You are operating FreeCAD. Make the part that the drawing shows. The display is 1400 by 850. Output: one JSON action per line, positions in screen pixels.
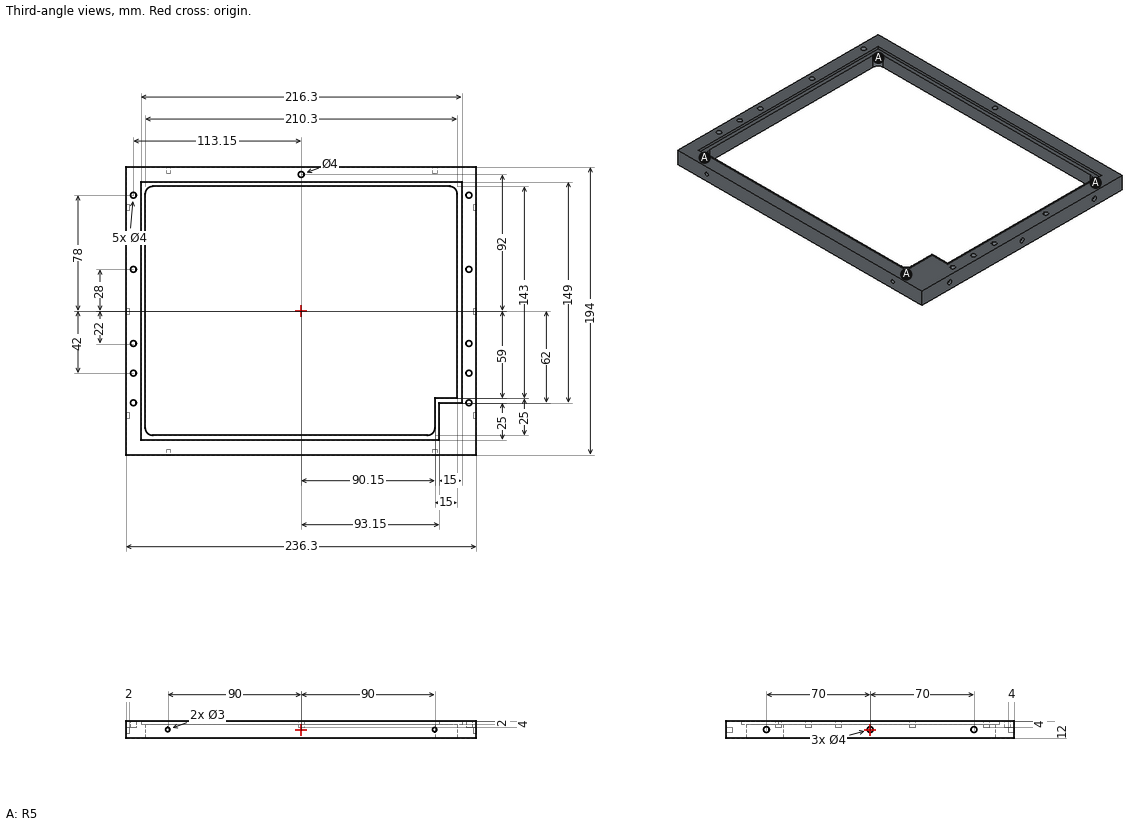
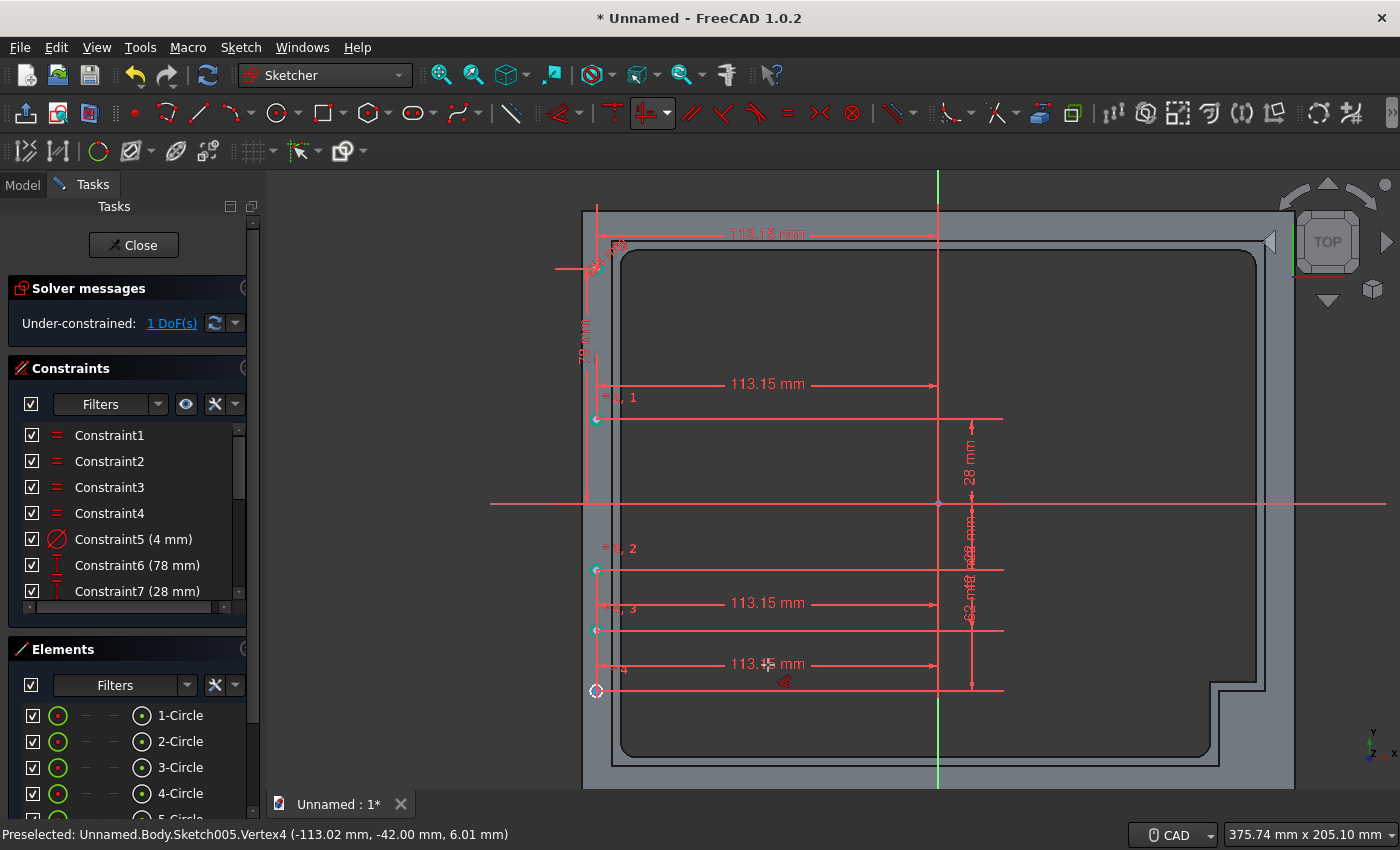
{"action": "left_click", "coordinate": [596, 691]}
{"action": "left_click", "coordinate": [767, 725]}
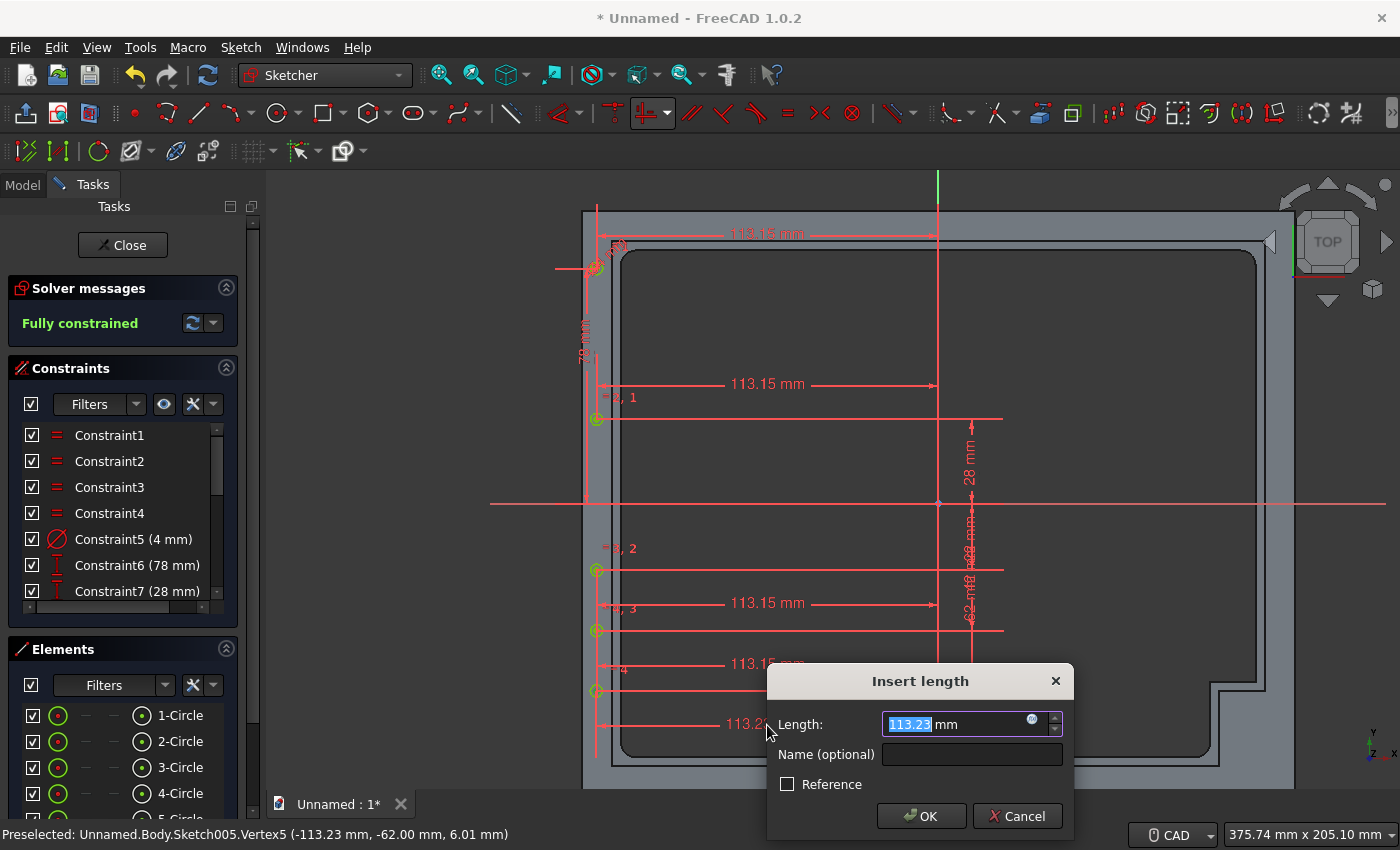
{"action": "type", "text": "113.15"}
{"action": "key", "text": "Return"}
{"action": "key", "text": "Escape"}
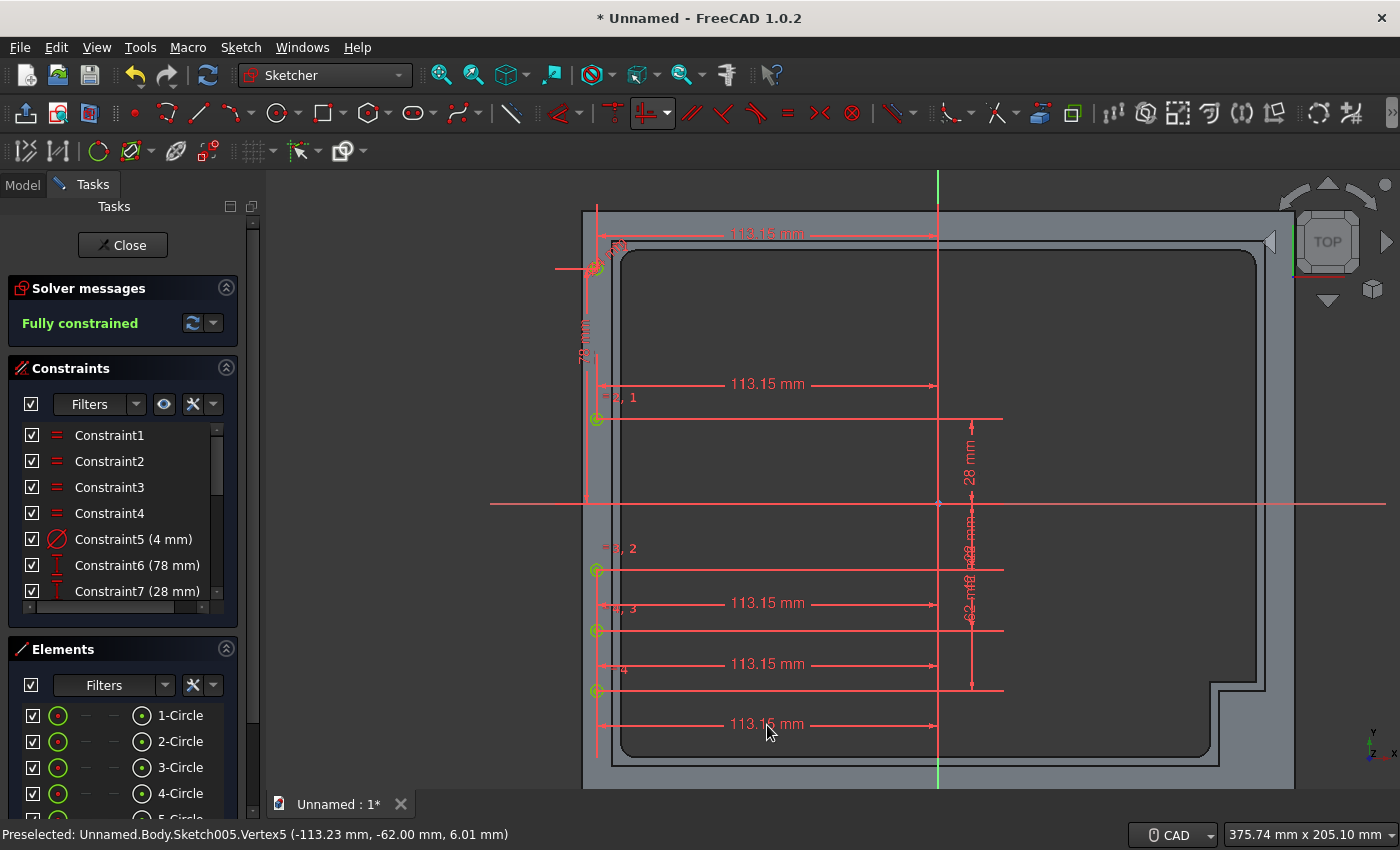
{"action": "left_click", "coordinate": [123, 245]}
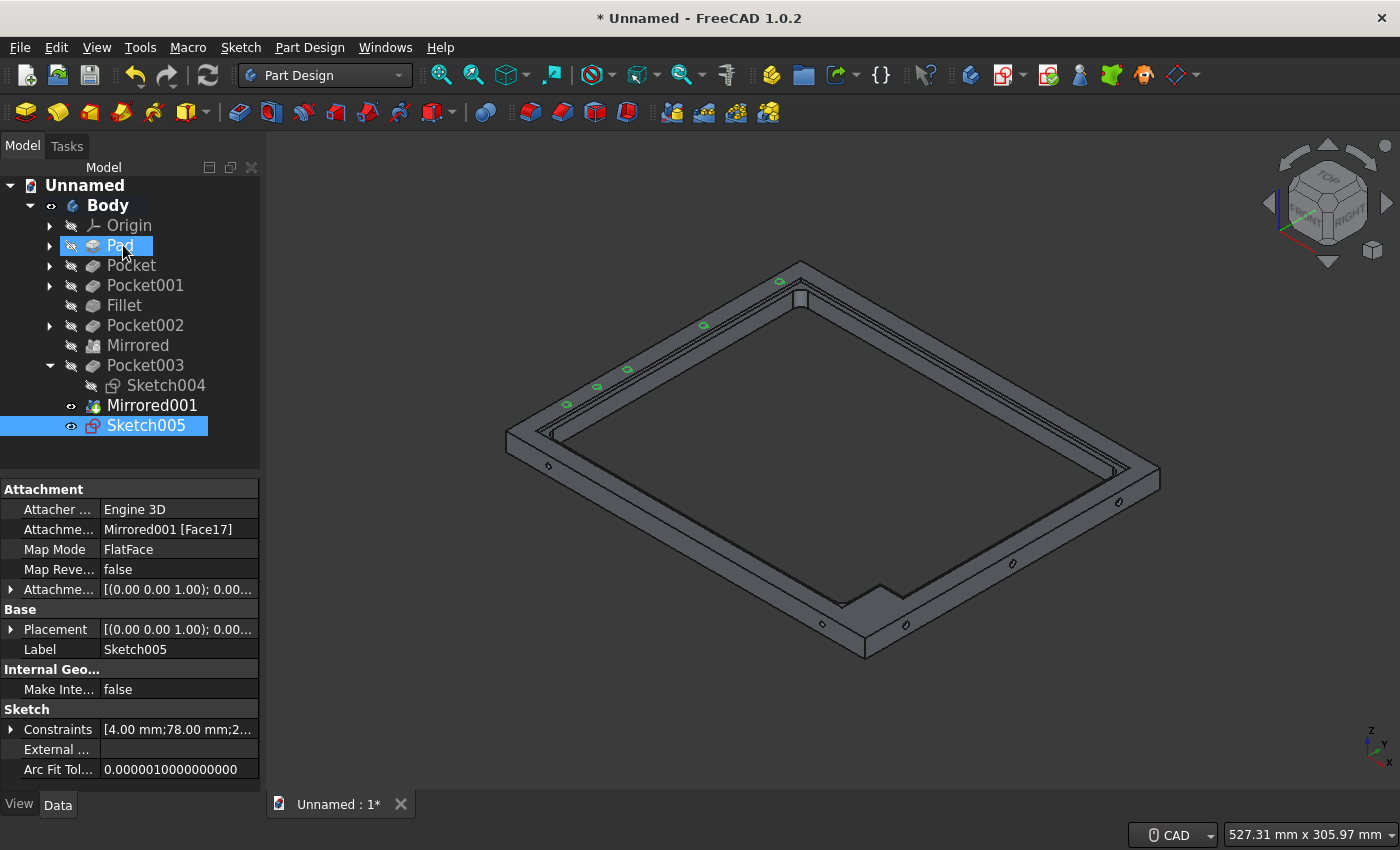
{"action": "left_click", "coordinate": [240, 112]}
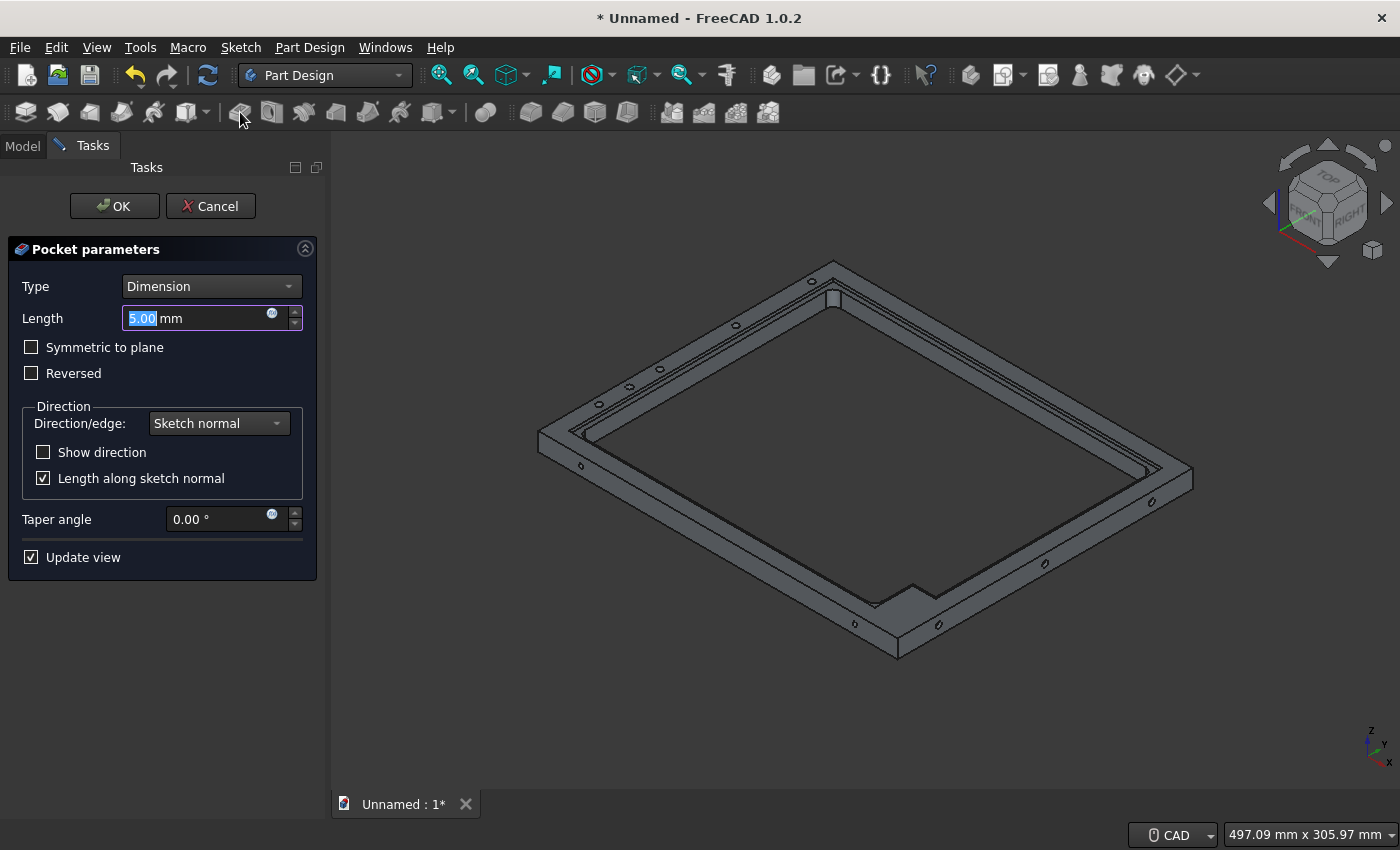
{"action": "type", "text": "4"}
{"action": "key", "text": "Tab"}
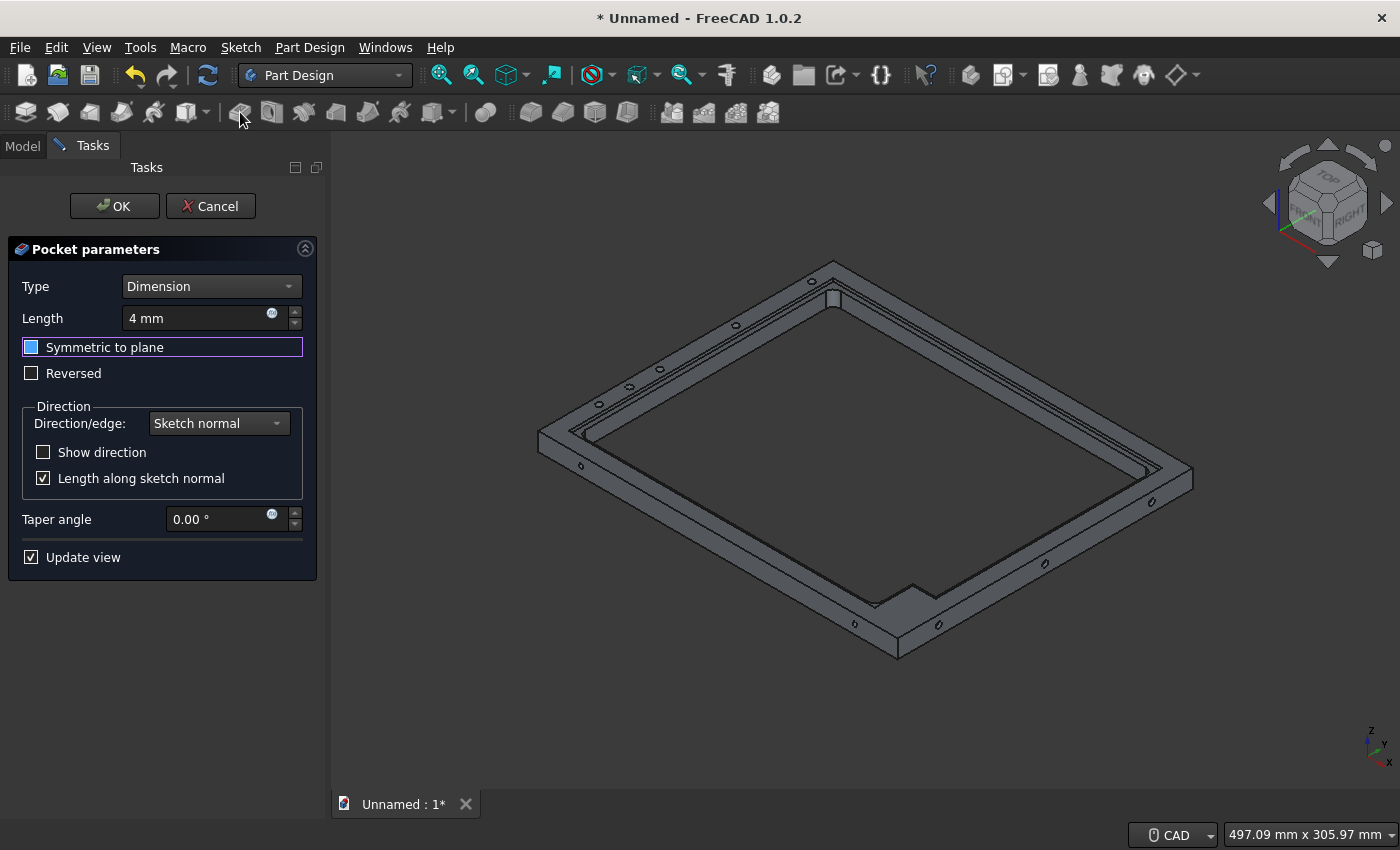
{"action": "left_click", "coordinate": [115, 206]}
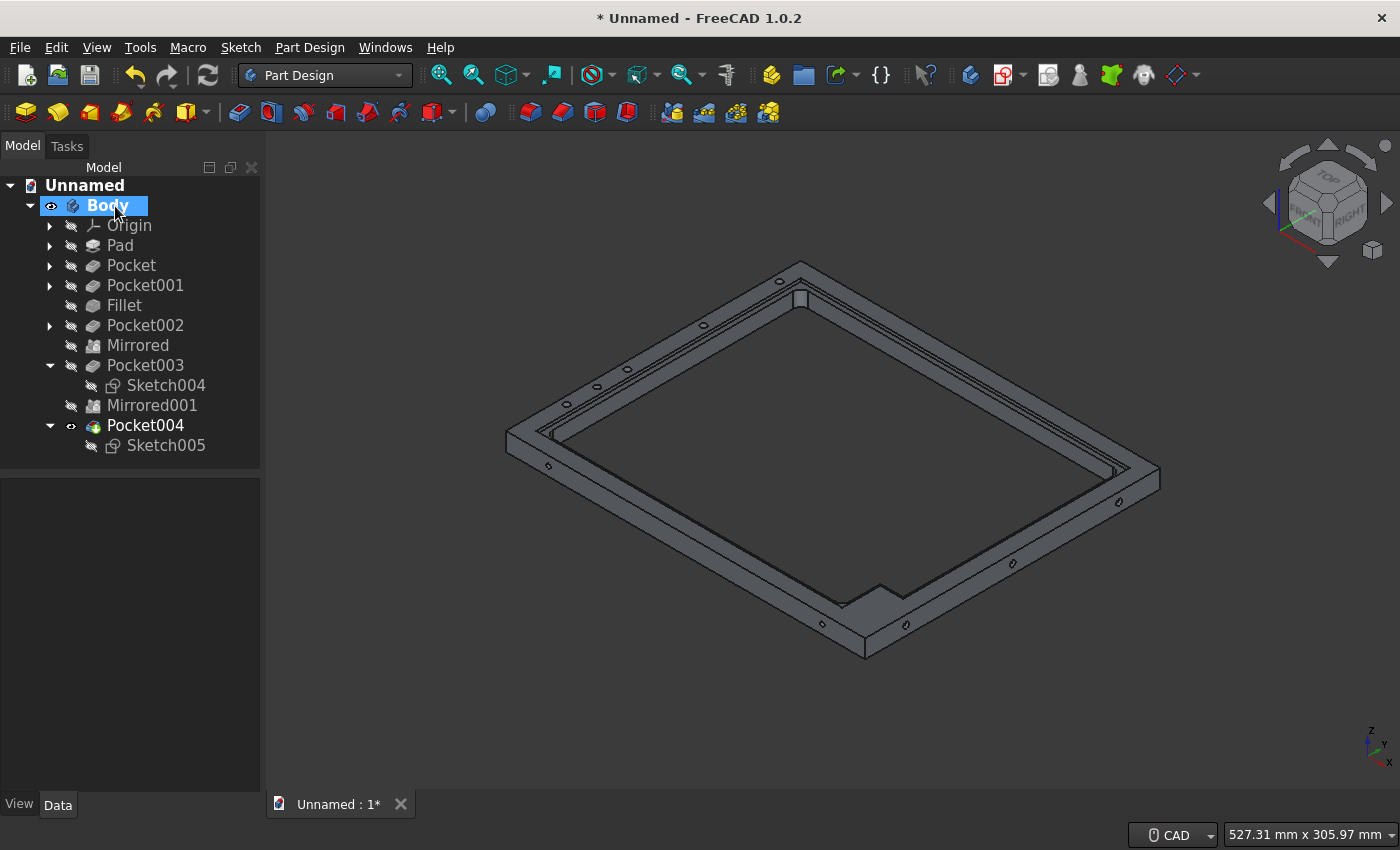
{"action": "left_click", "coordinate": [116, 426]}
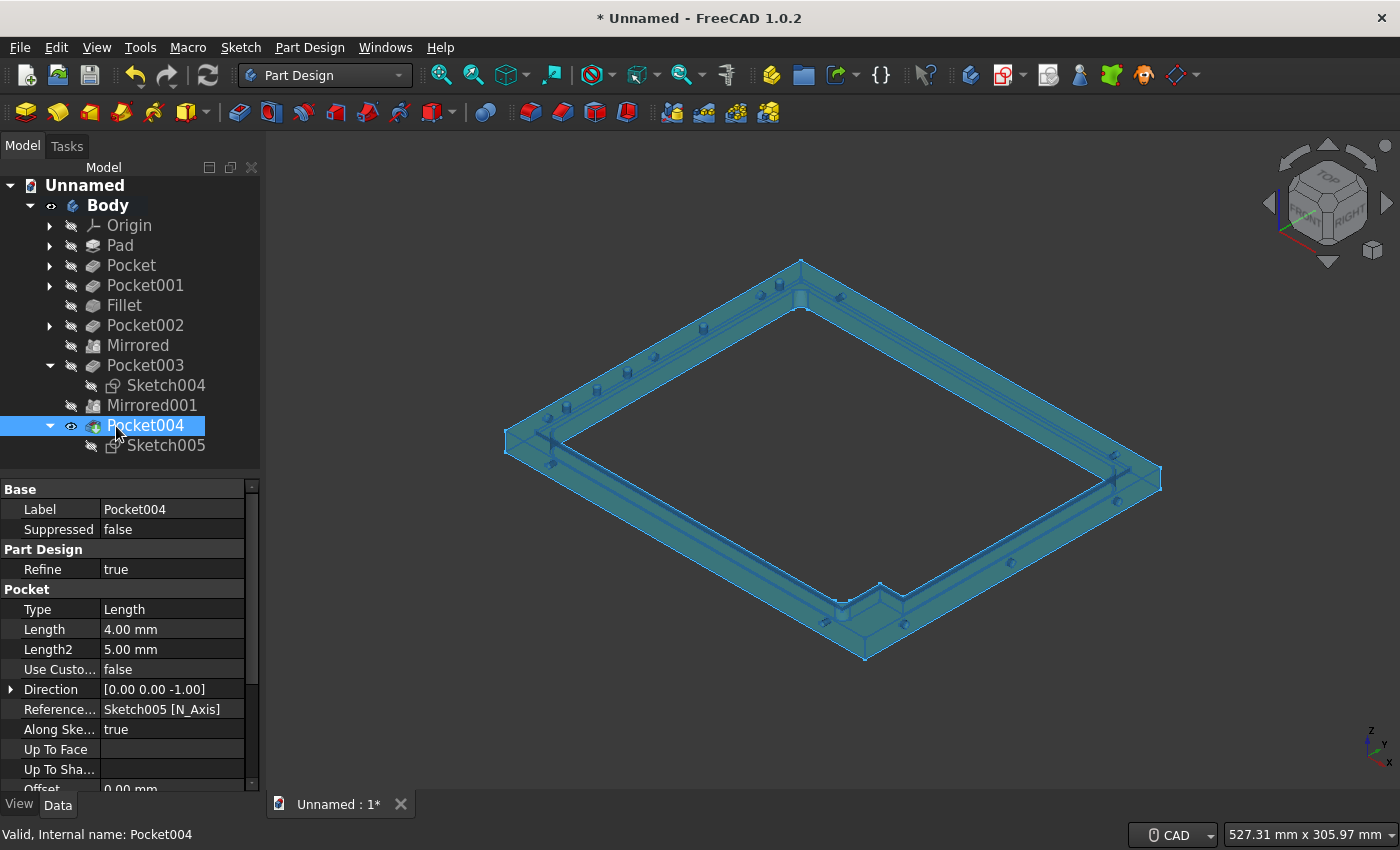
{"action": "left_click", "coordinate": [672, 112]}